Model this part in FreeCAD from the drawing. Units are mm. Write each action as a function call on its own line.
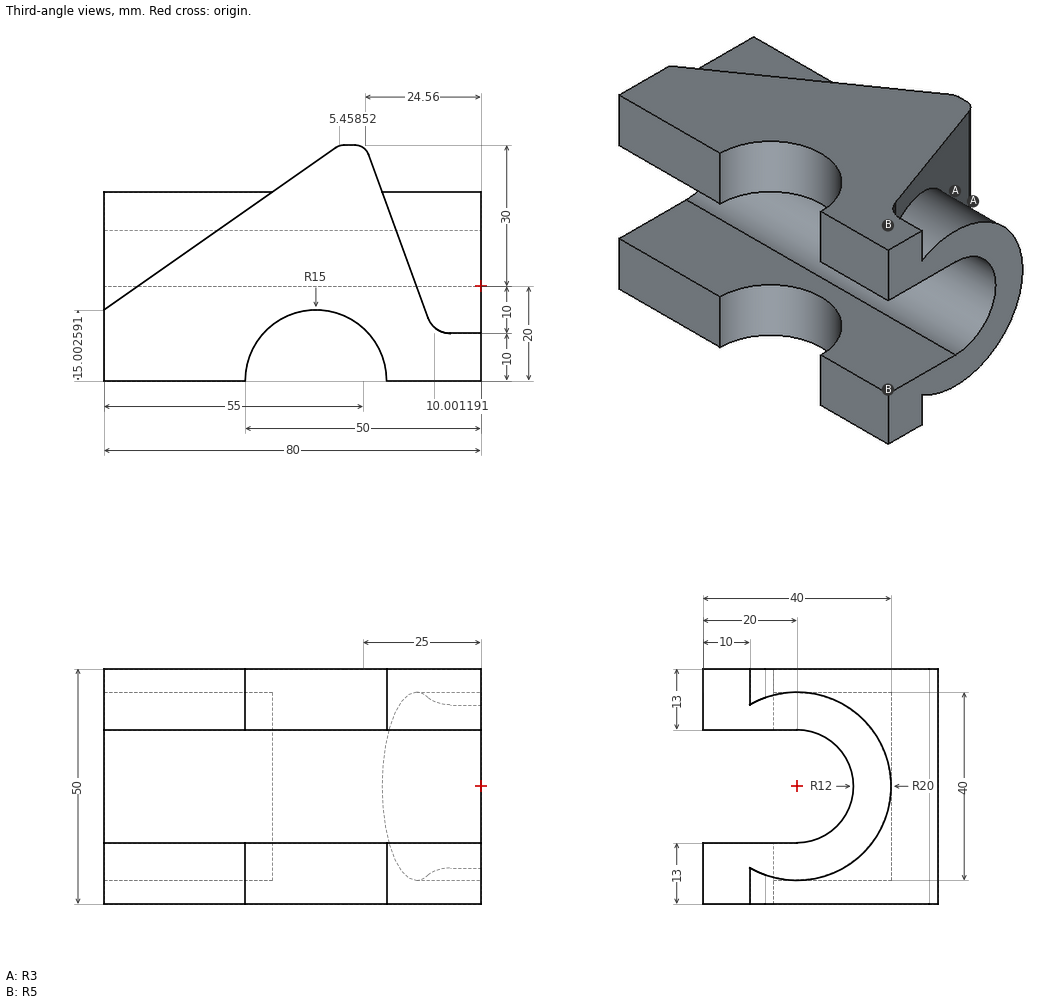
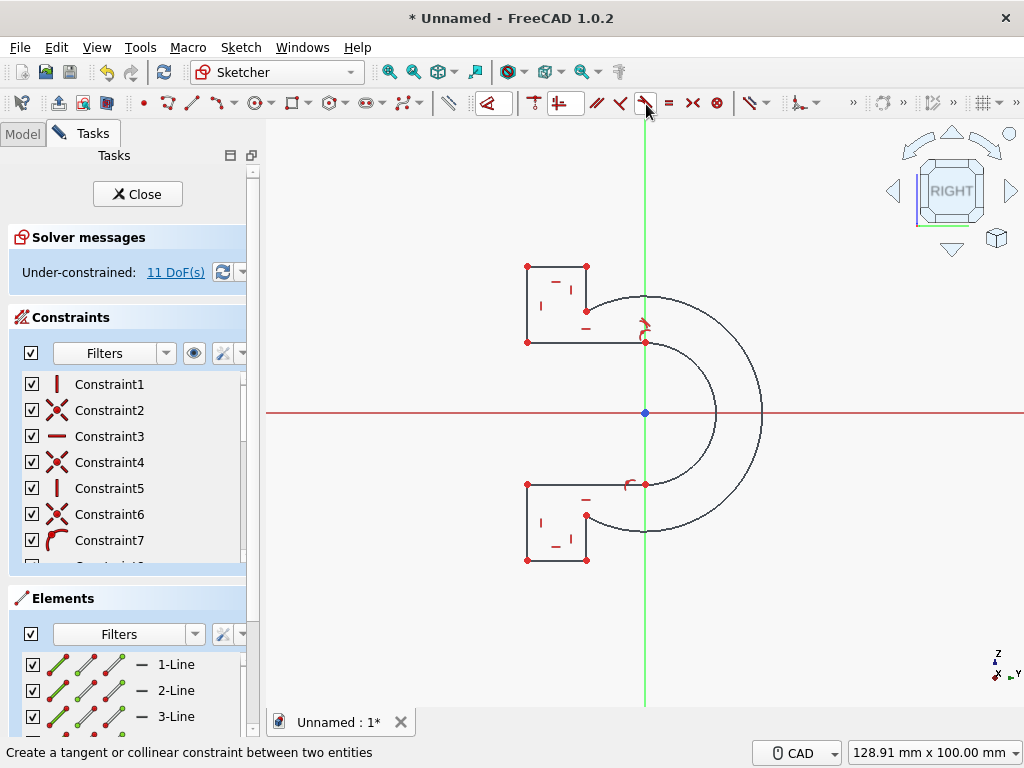
click(702, 456)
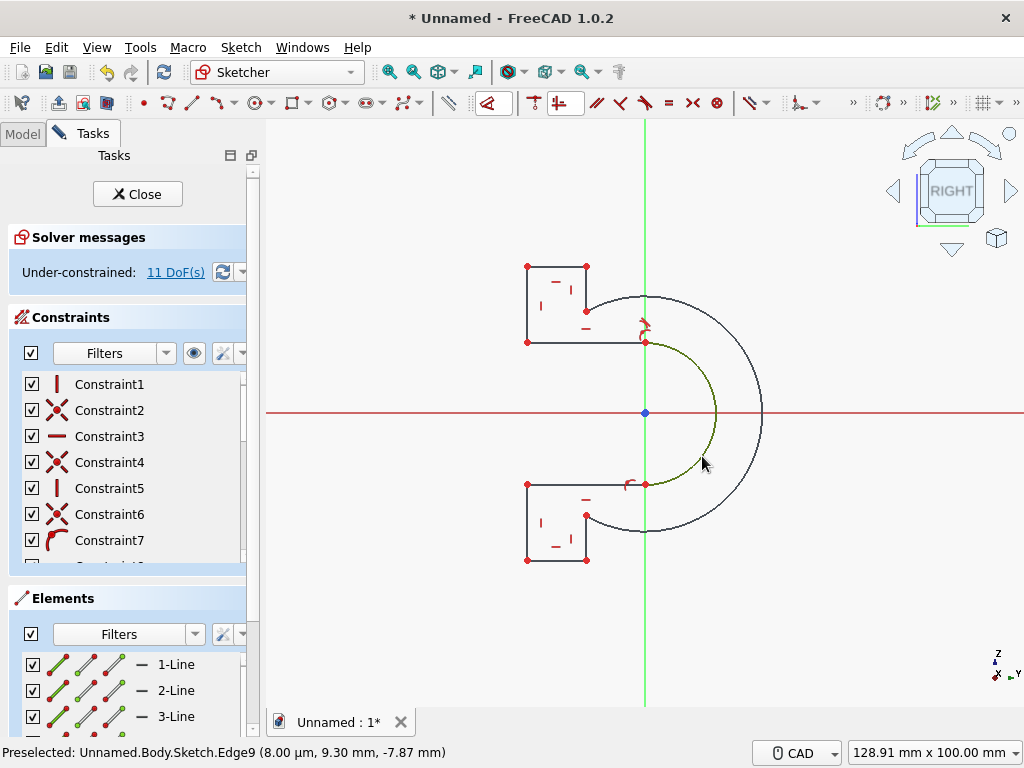
click(723, 501)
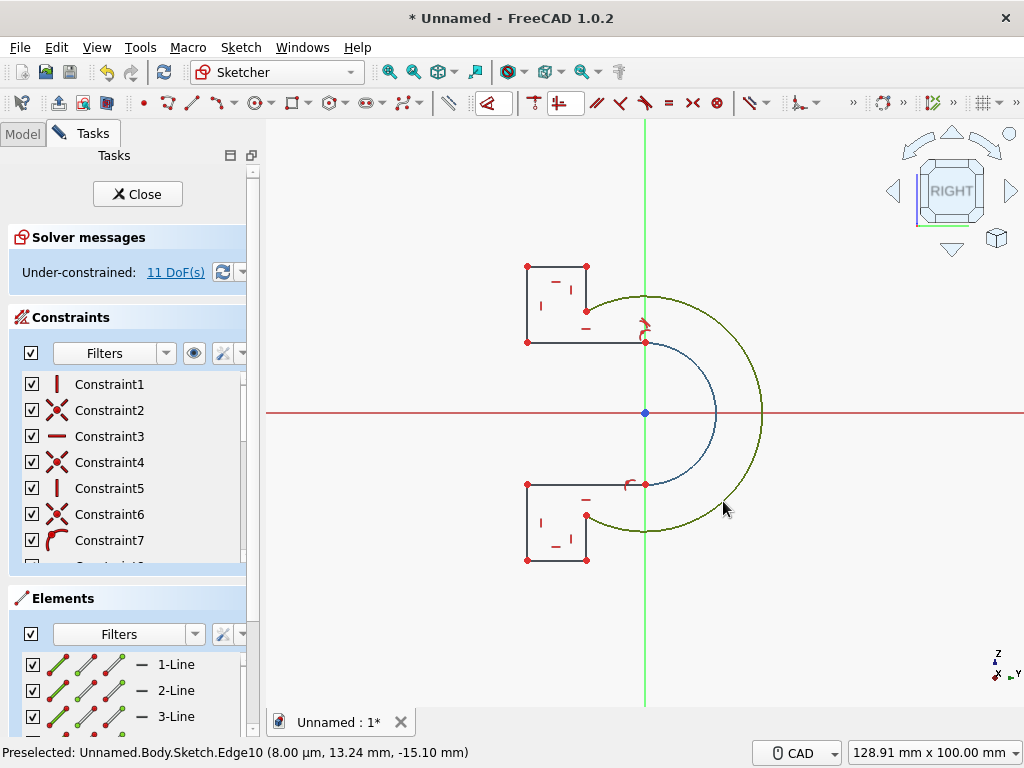
click(534, 104)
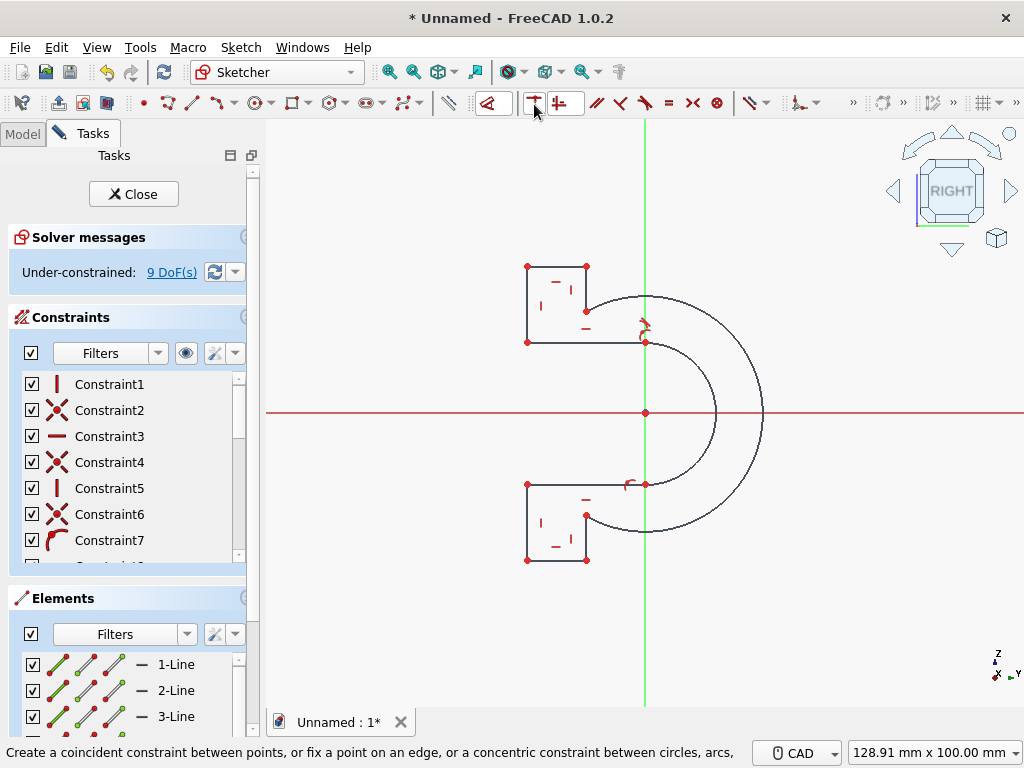
click(645, 414)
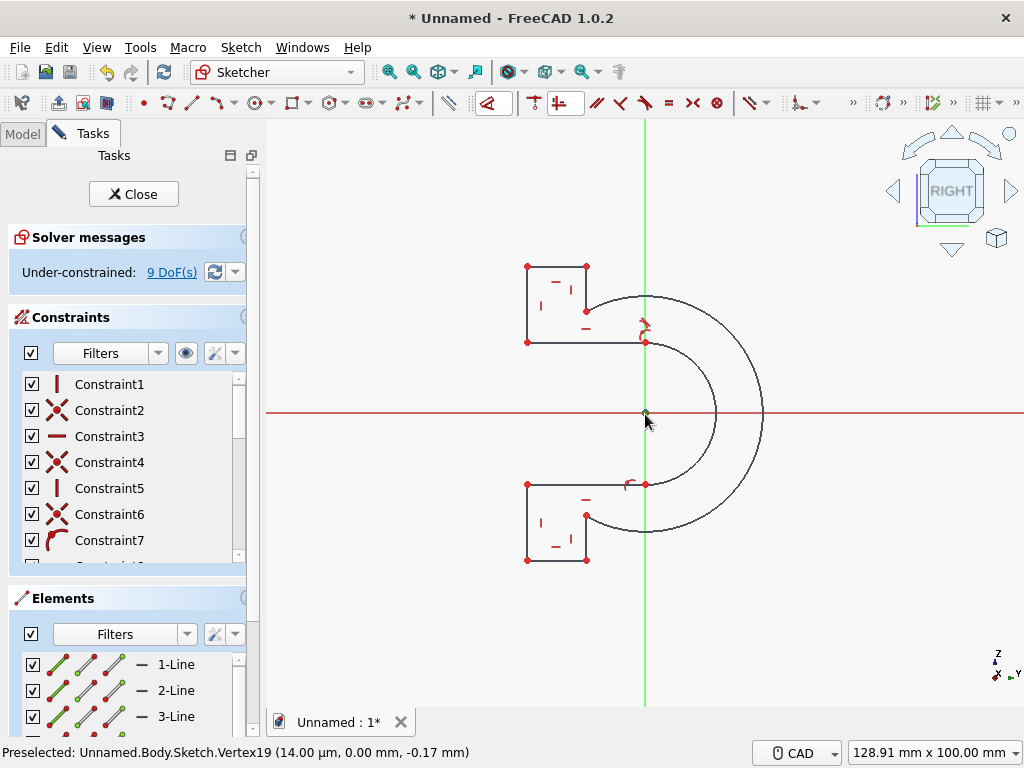
click(334, 413)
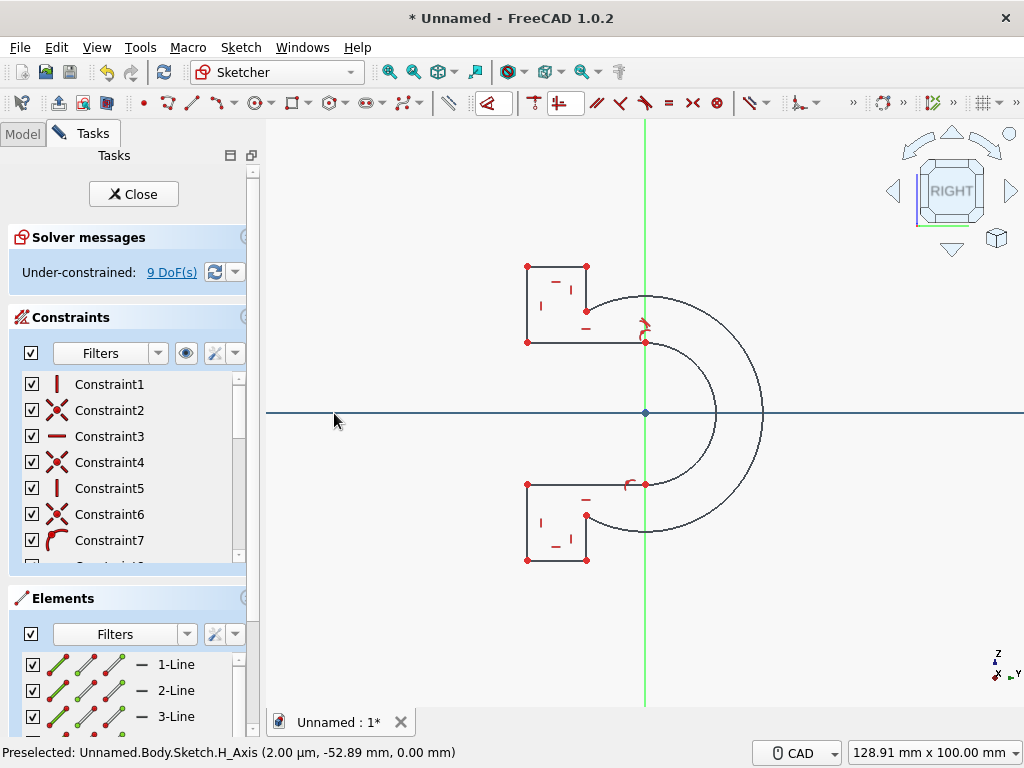
click(534, 104)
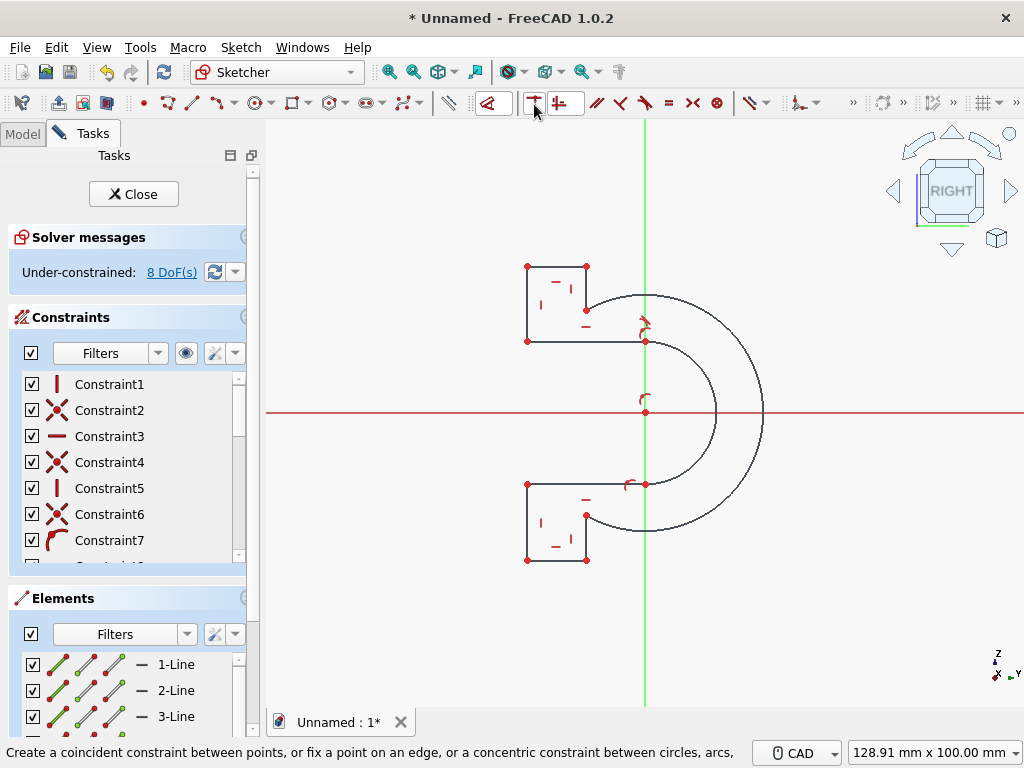
key(d)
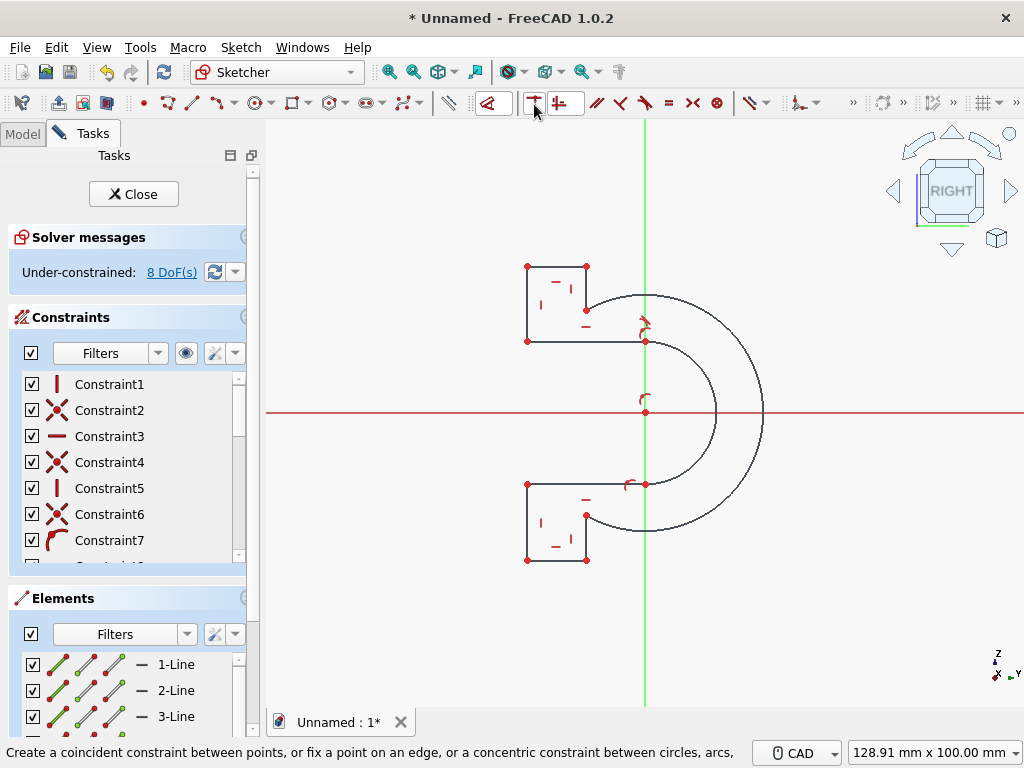
click(703, 455)
click(729, 474)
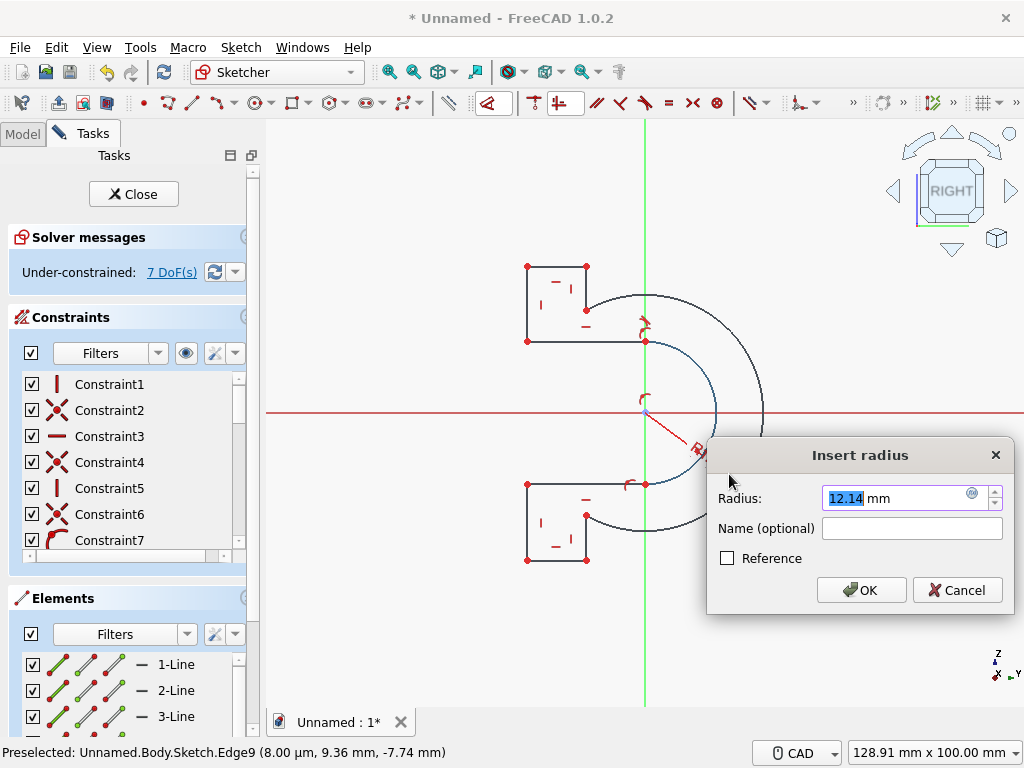
text(12)
key(Return)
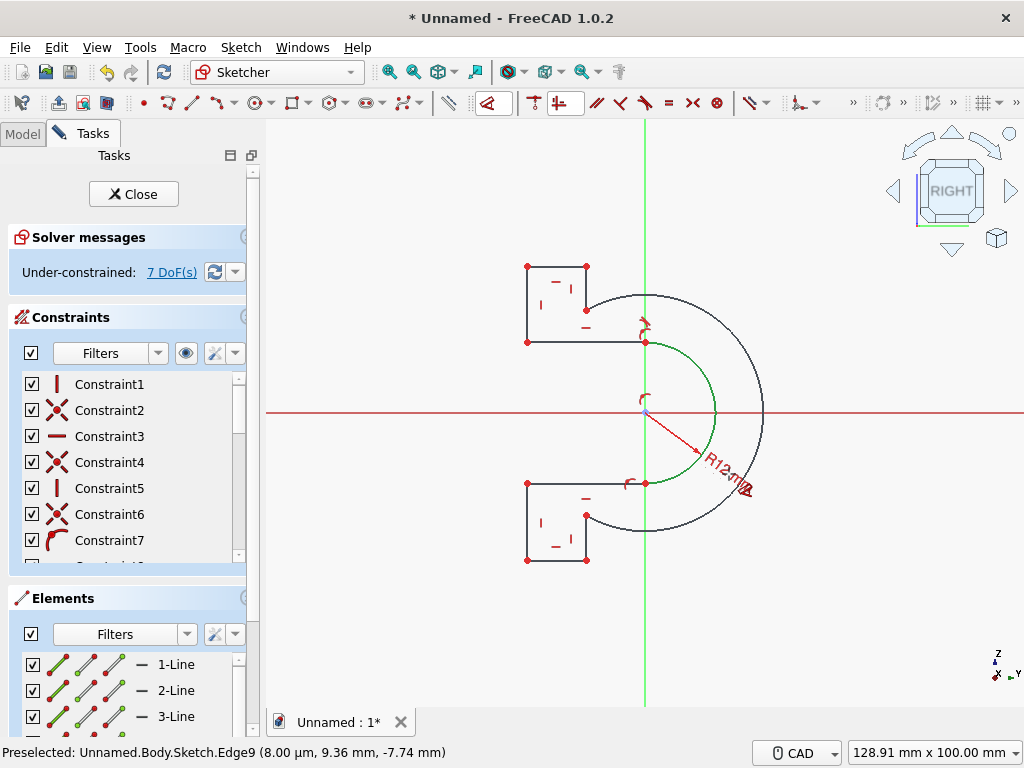
click(724, 501)
click(745, 525)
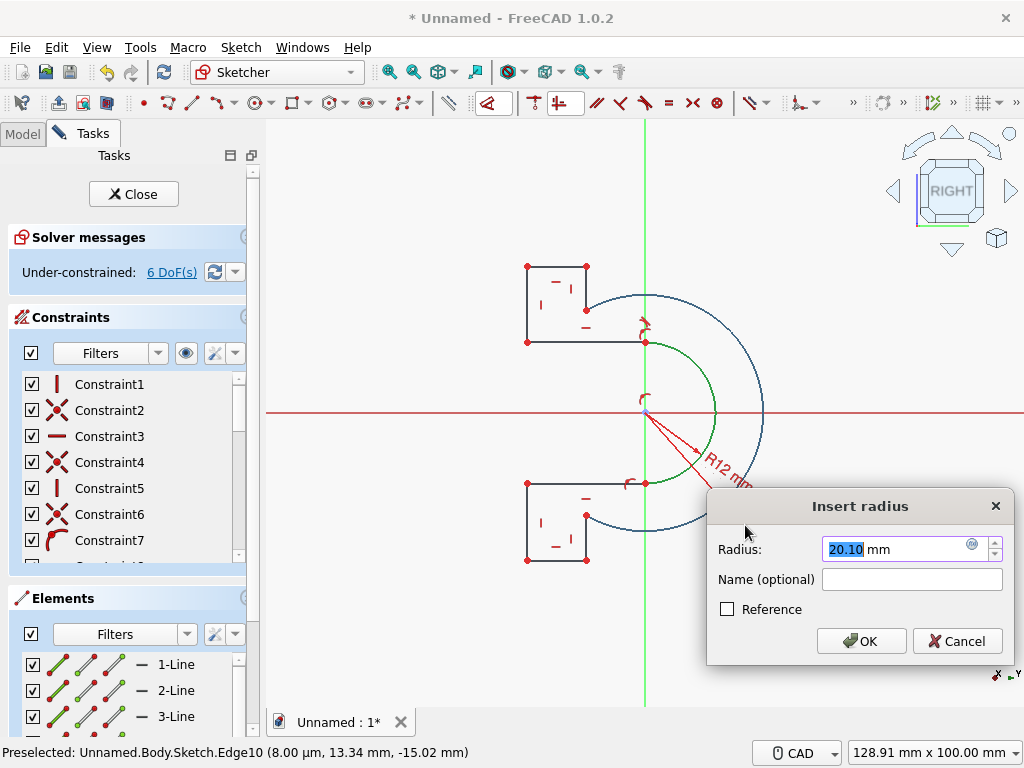
text(20)
key(Return)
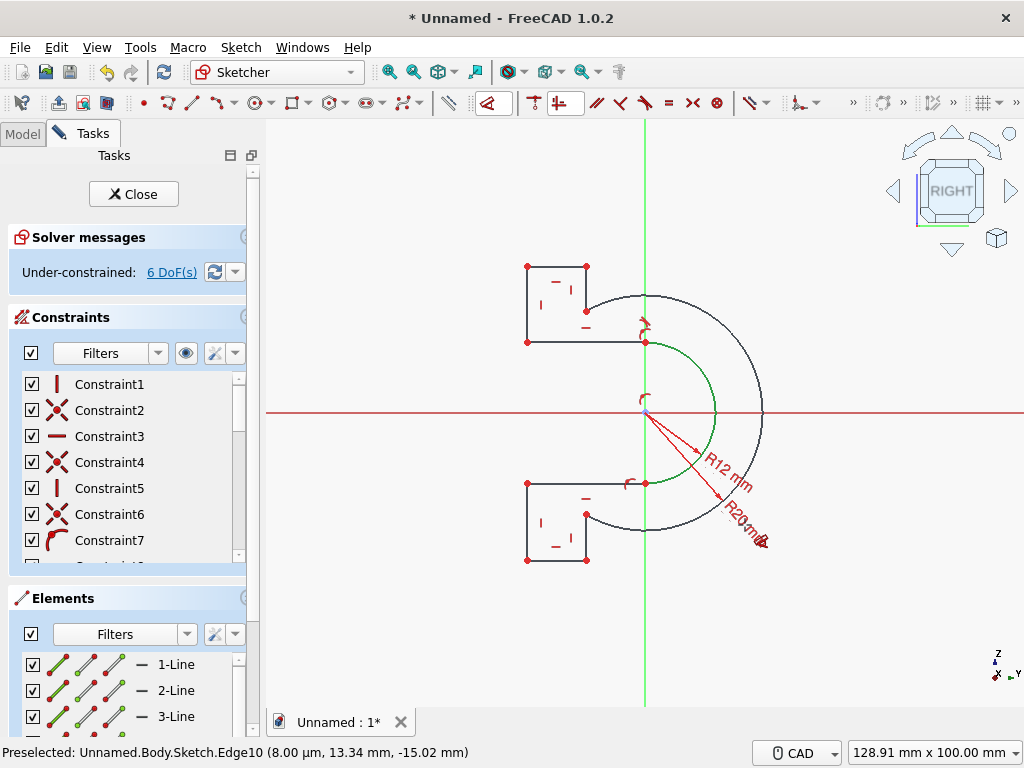
click(568, 267)
click(557, 233)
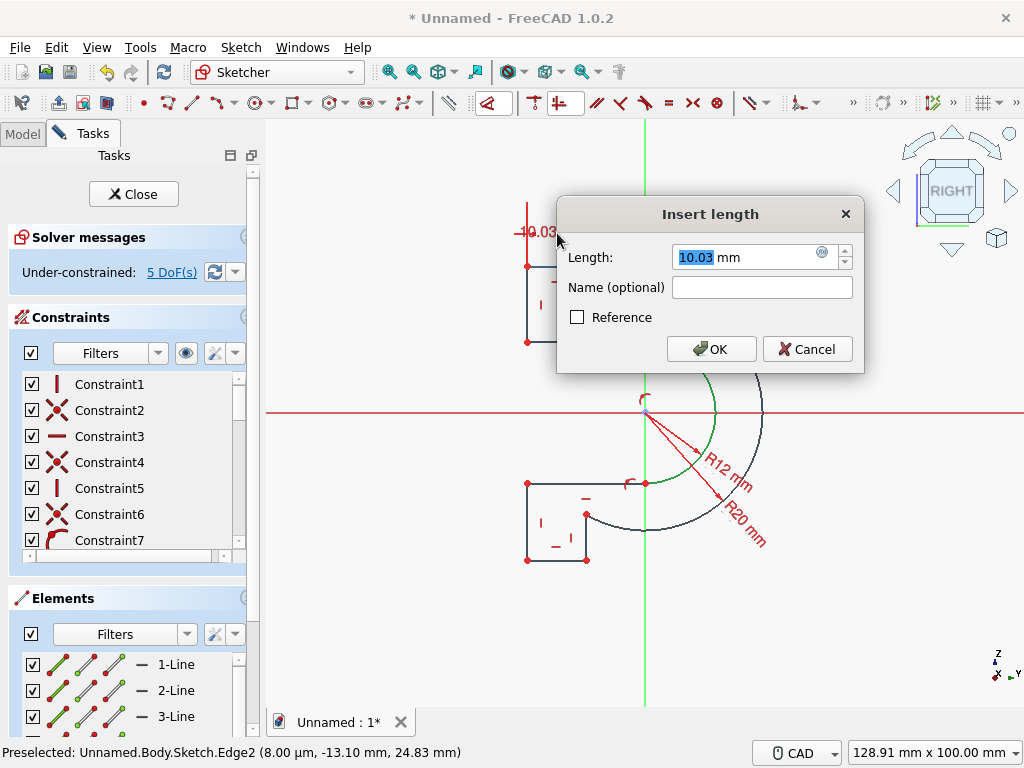
text(10)
key(Return)